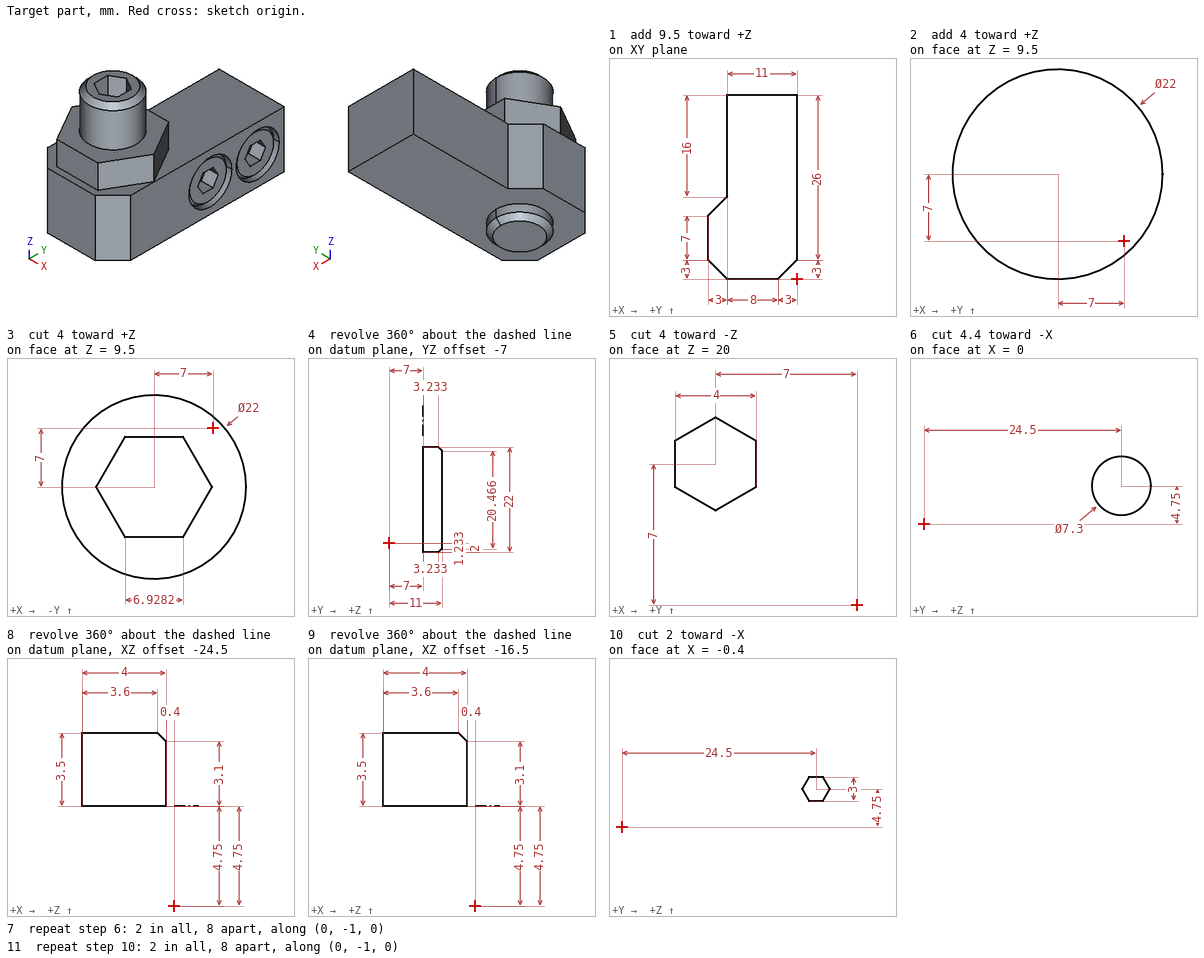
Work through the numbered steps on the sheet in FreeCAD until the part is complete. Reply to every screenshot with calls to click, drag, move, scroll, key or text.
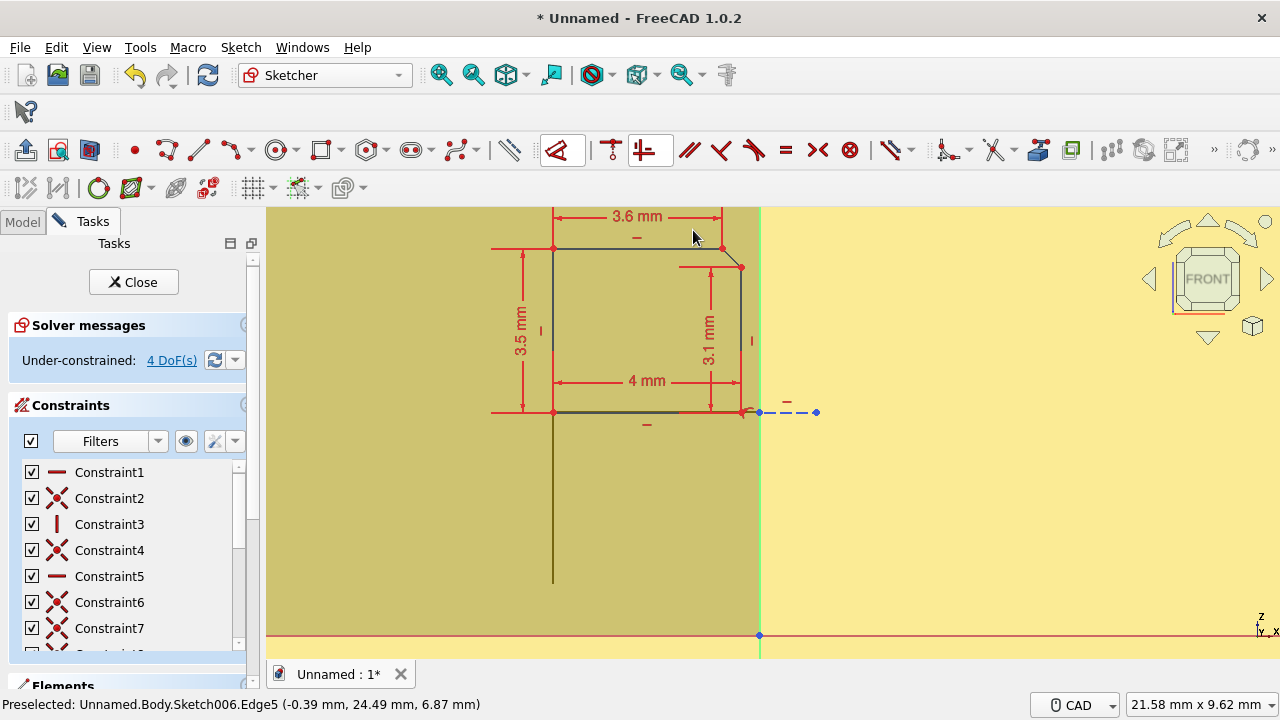
scroll(741, 413, up, 4)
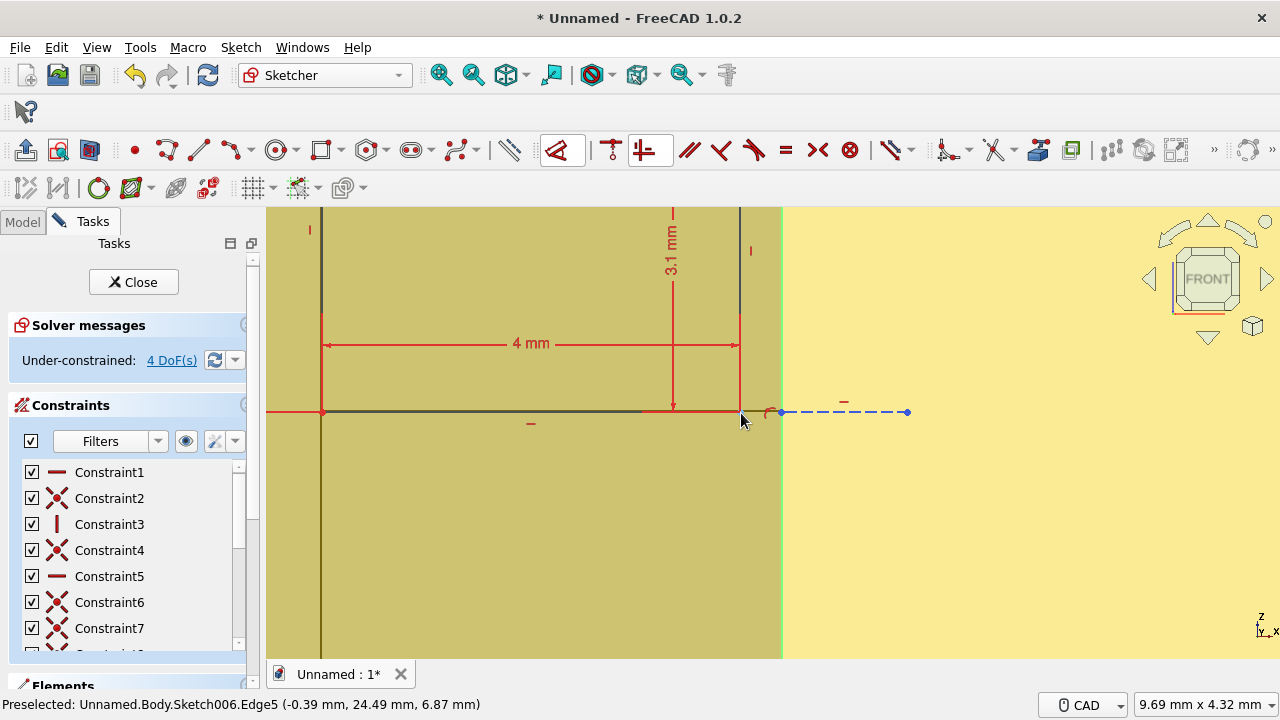
click(740, 412)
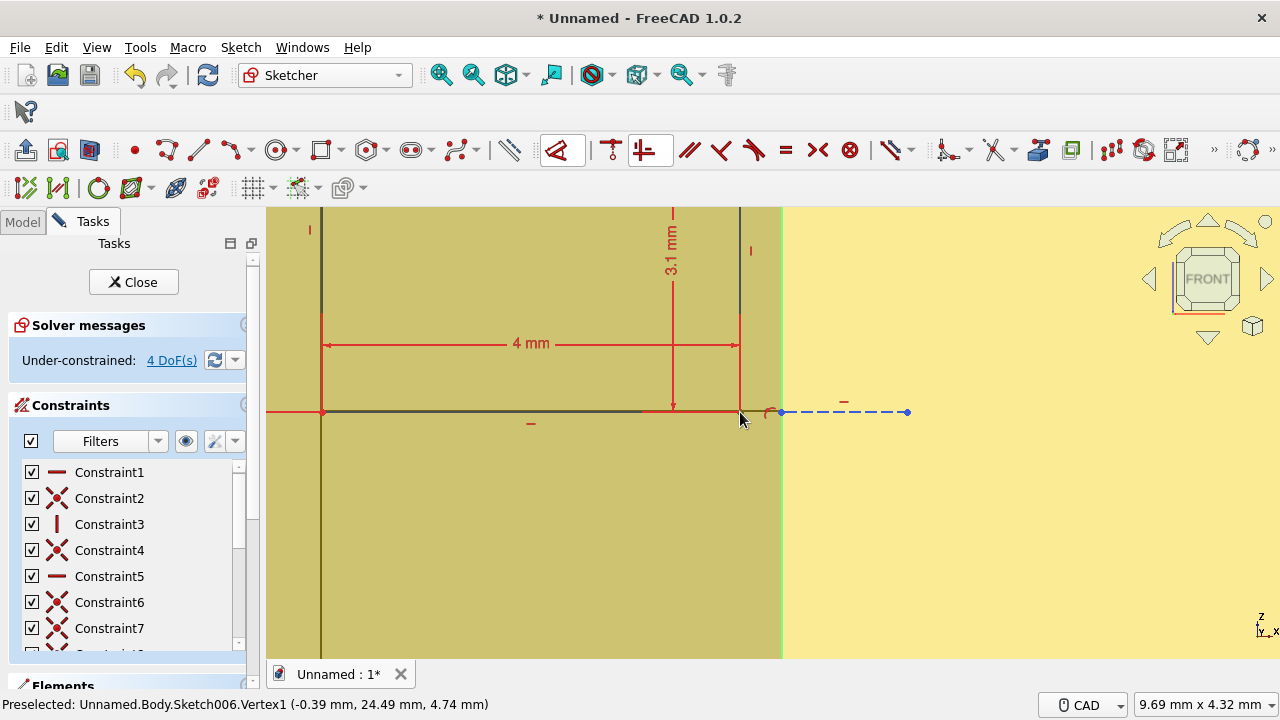
key(l)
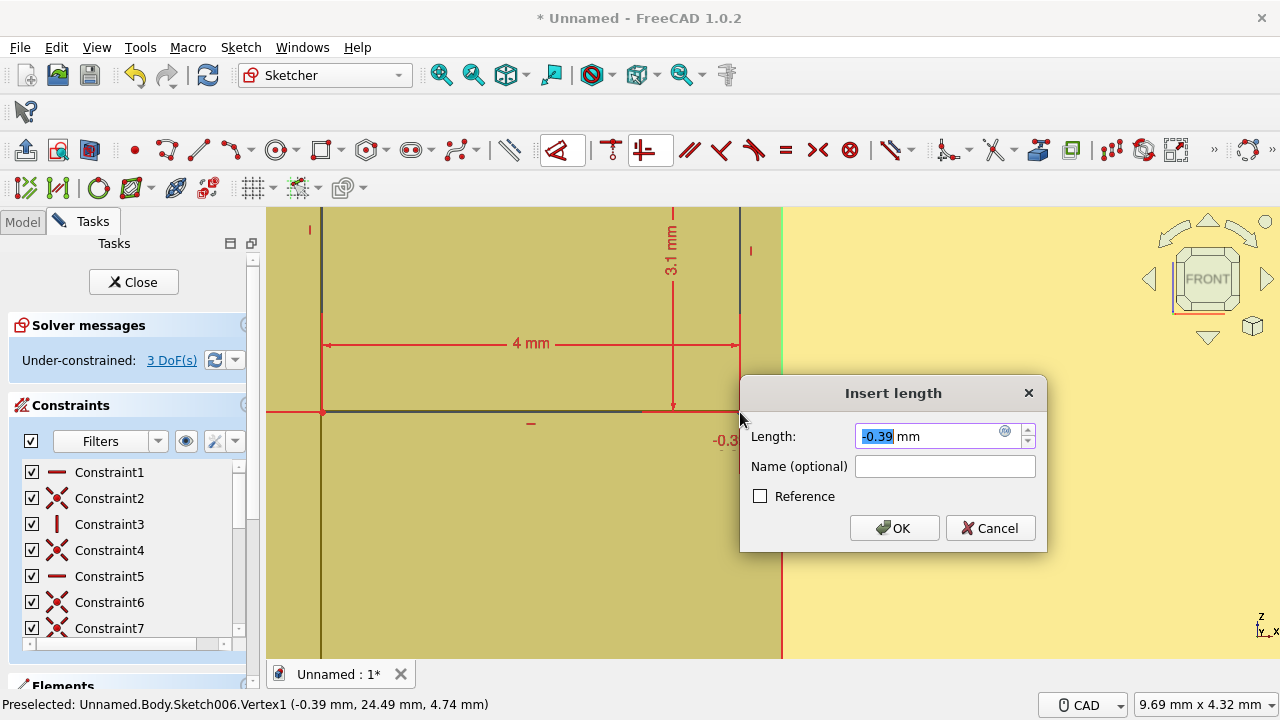
text(-0.4)
key(Return)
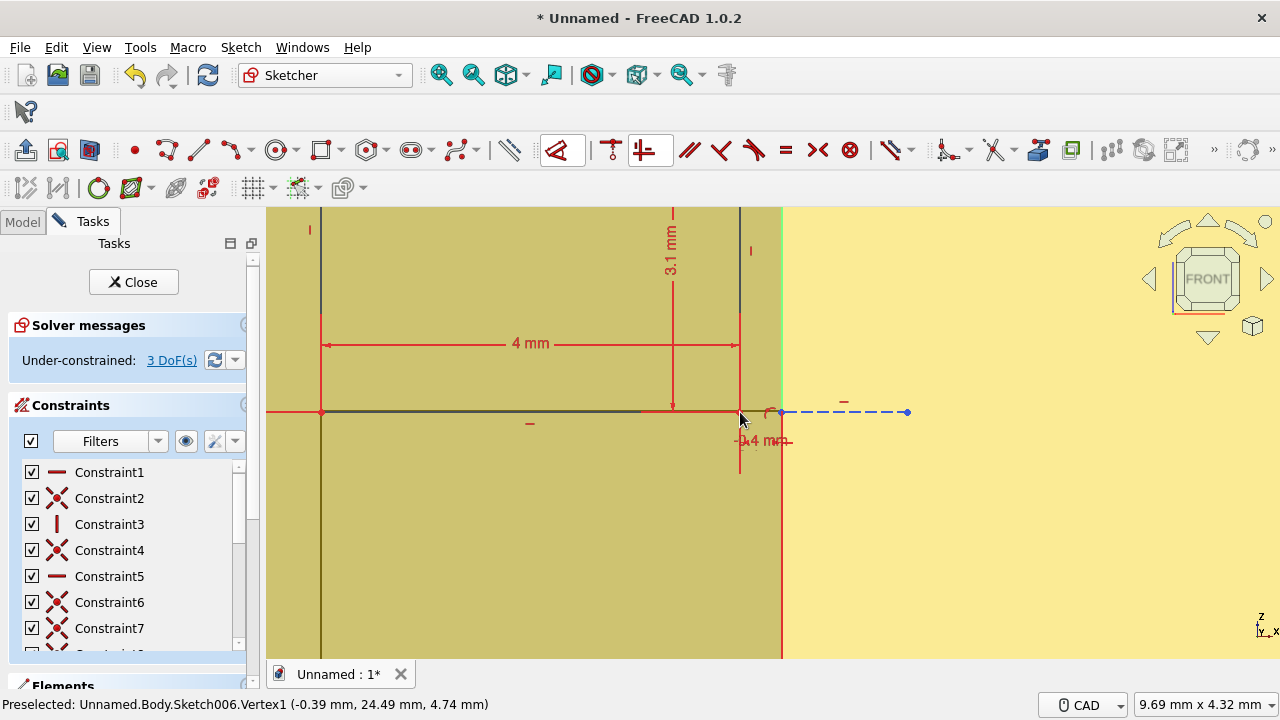
click(740, 412)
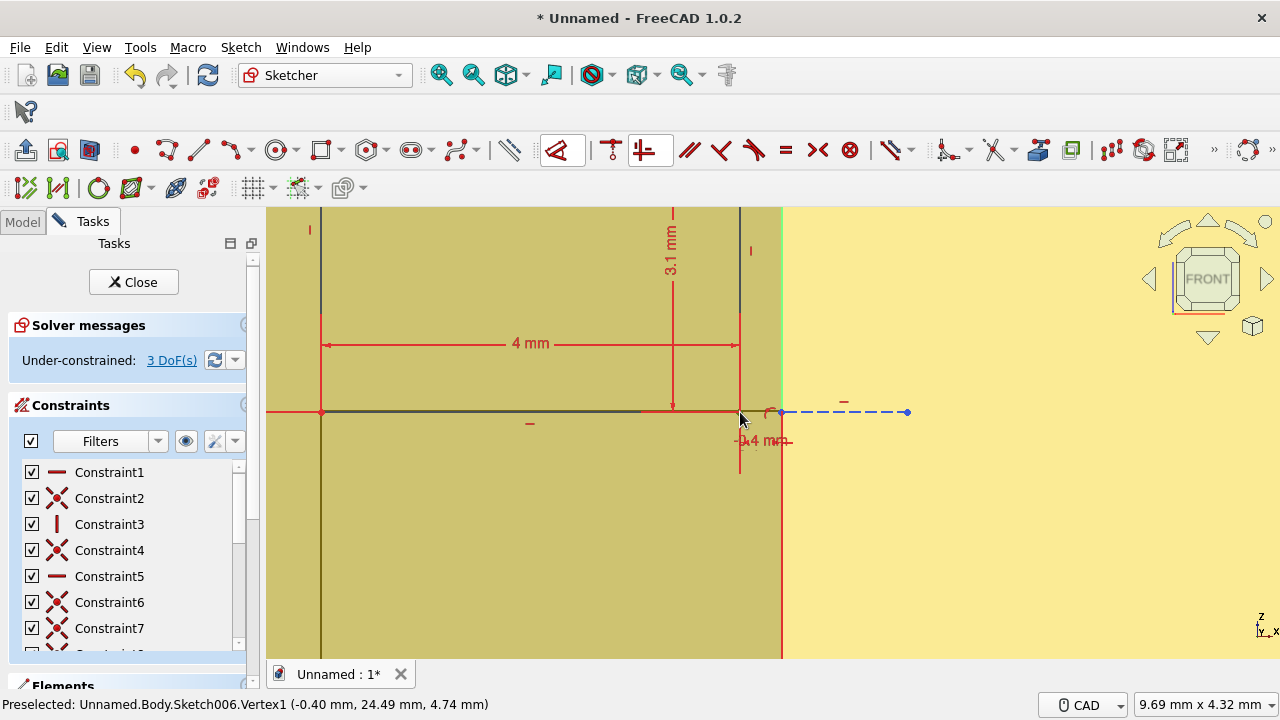
key(i)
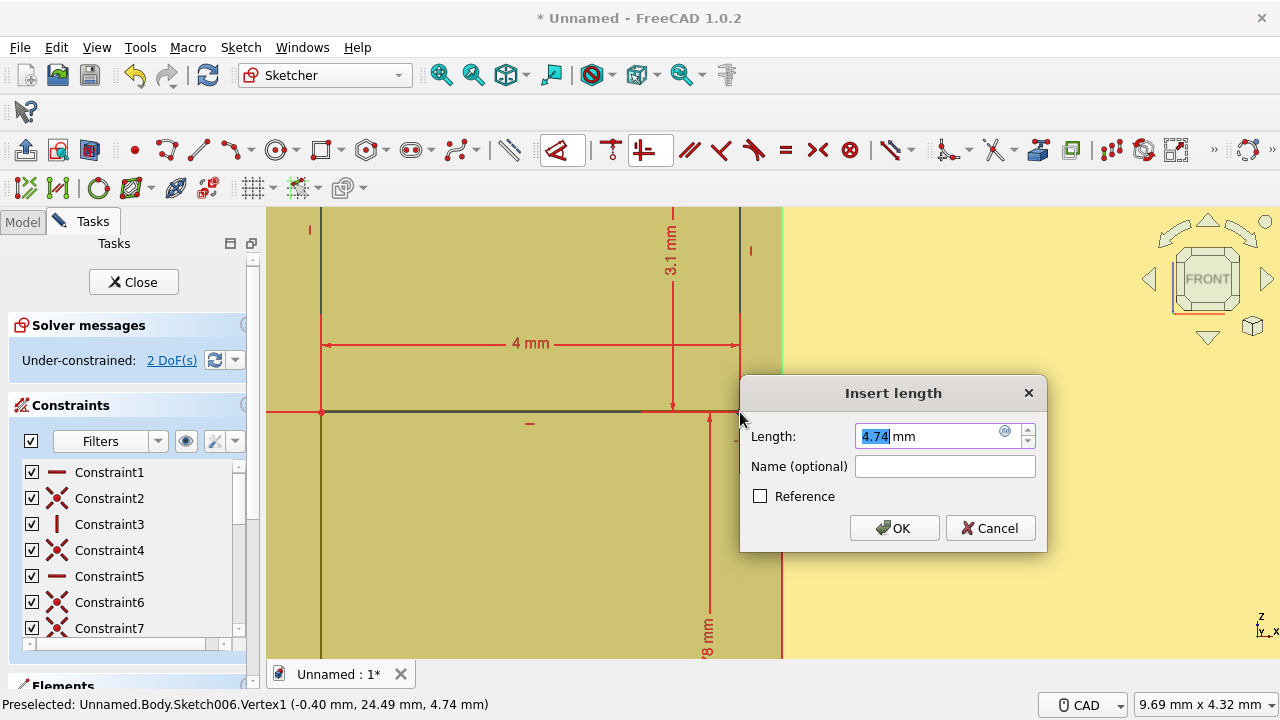
text(4.75)
key(Return)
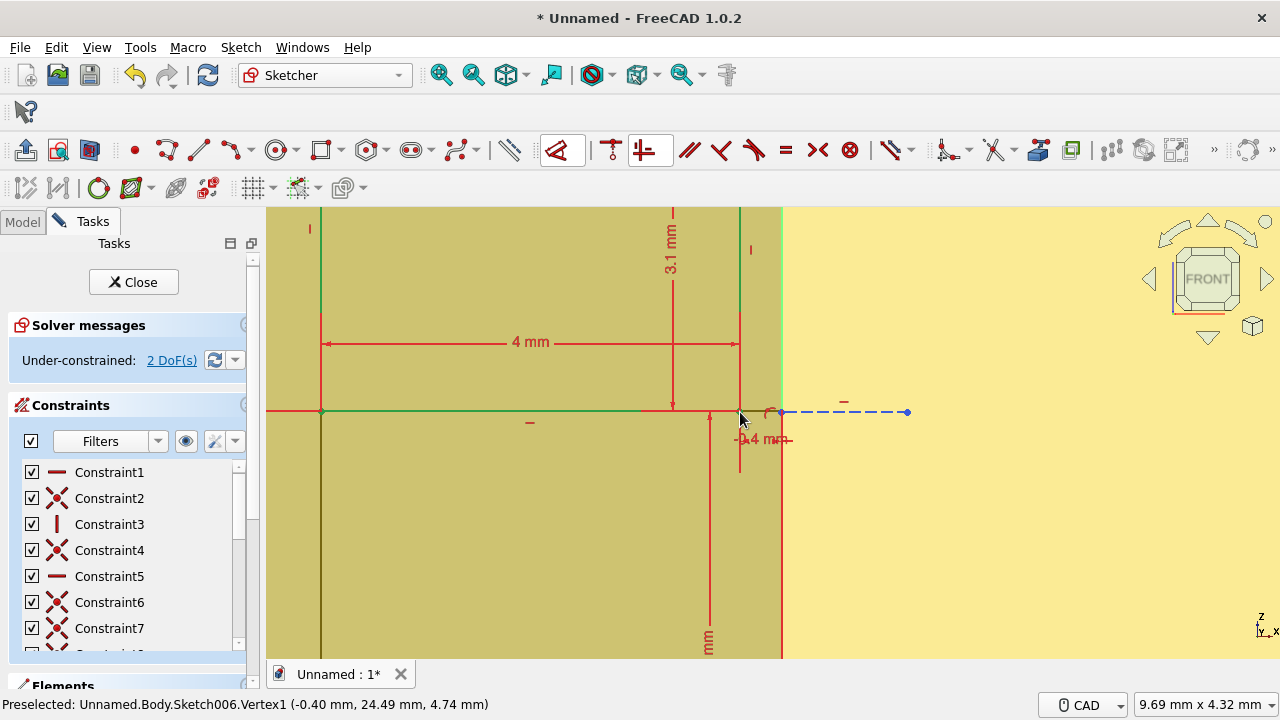
click(782, 412)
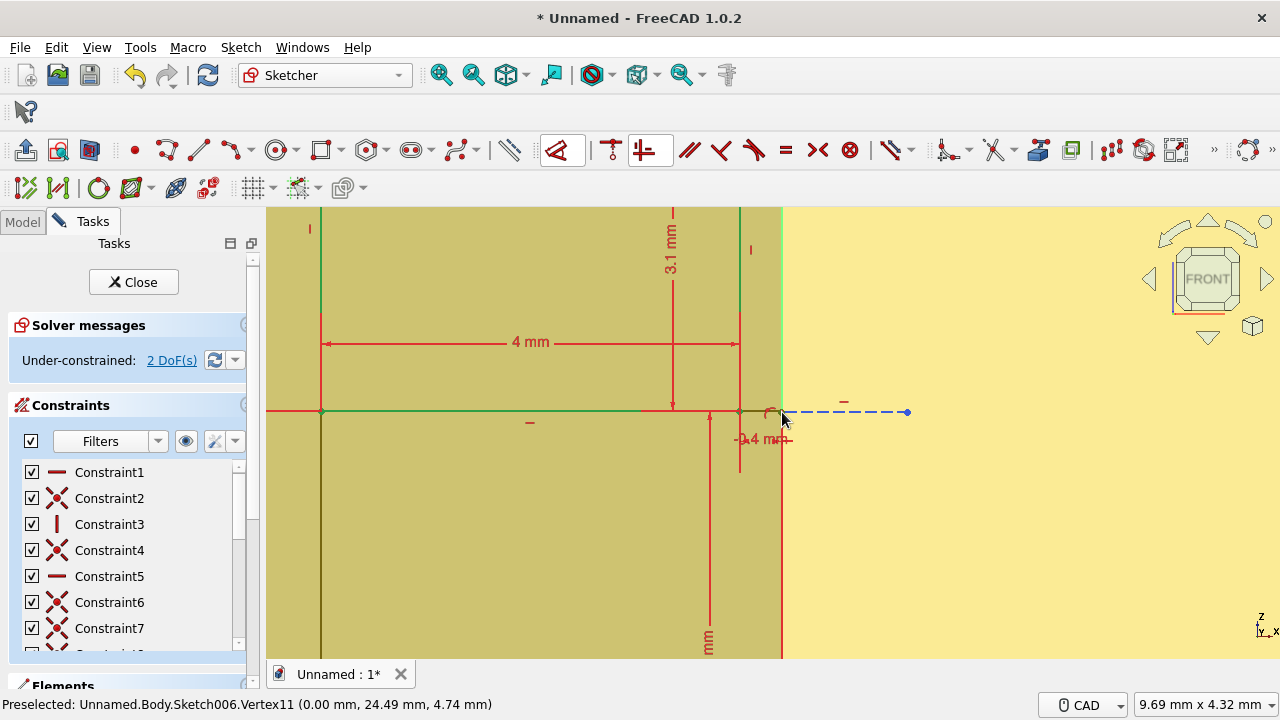
click(580, 150)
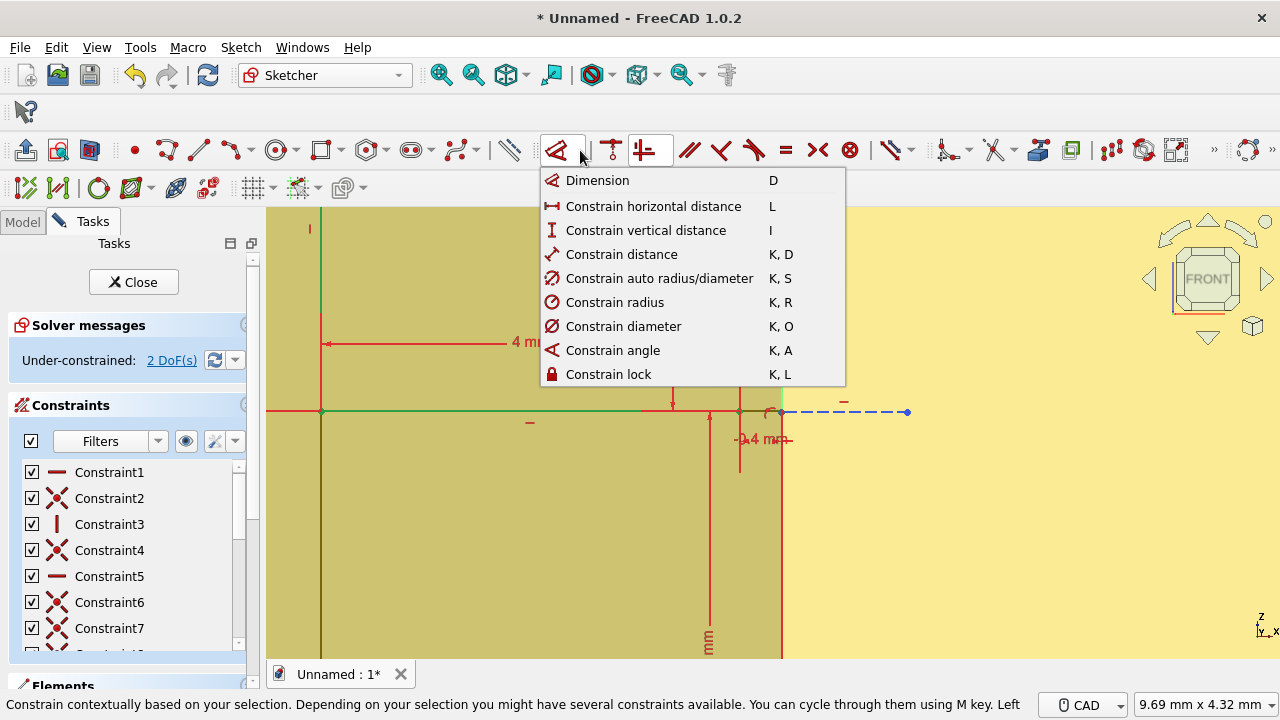
click(693, 230)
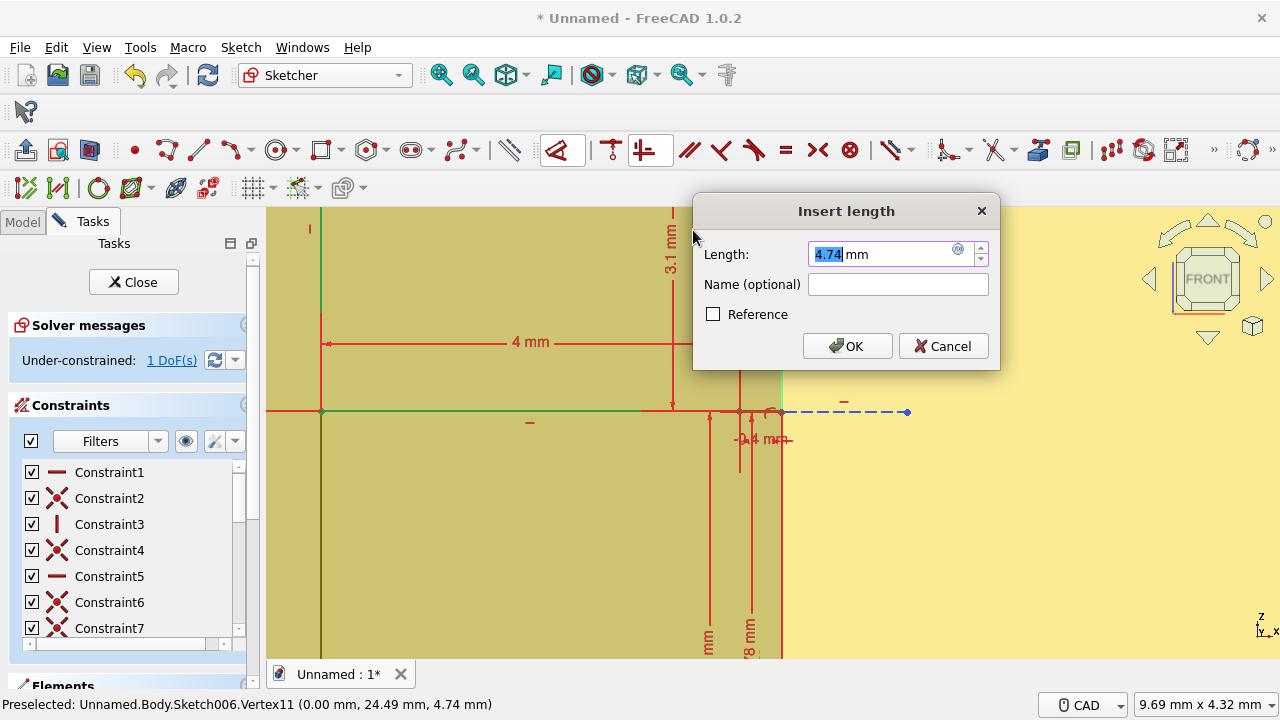
text(4.75)
key(Return)